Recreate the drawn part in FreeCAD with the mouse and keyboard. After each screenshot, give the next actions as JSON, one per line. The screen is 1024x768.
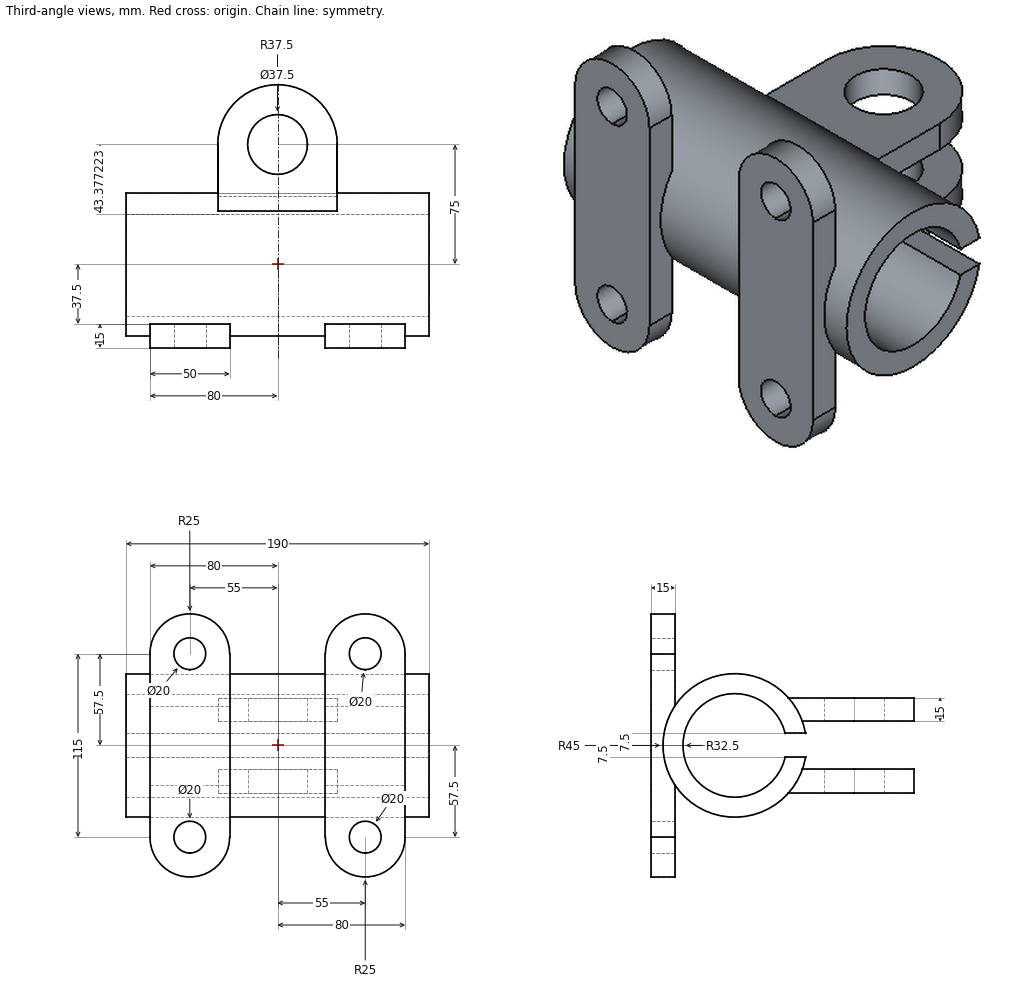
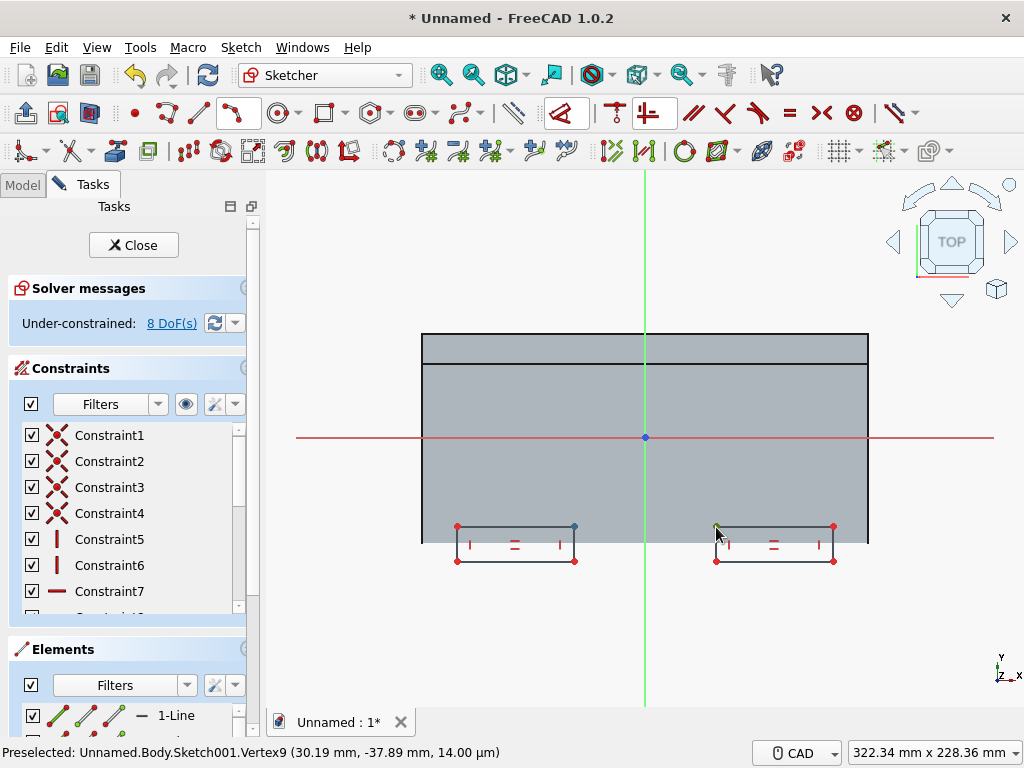
{"action": "left_click", "coordinate": [645, 645]}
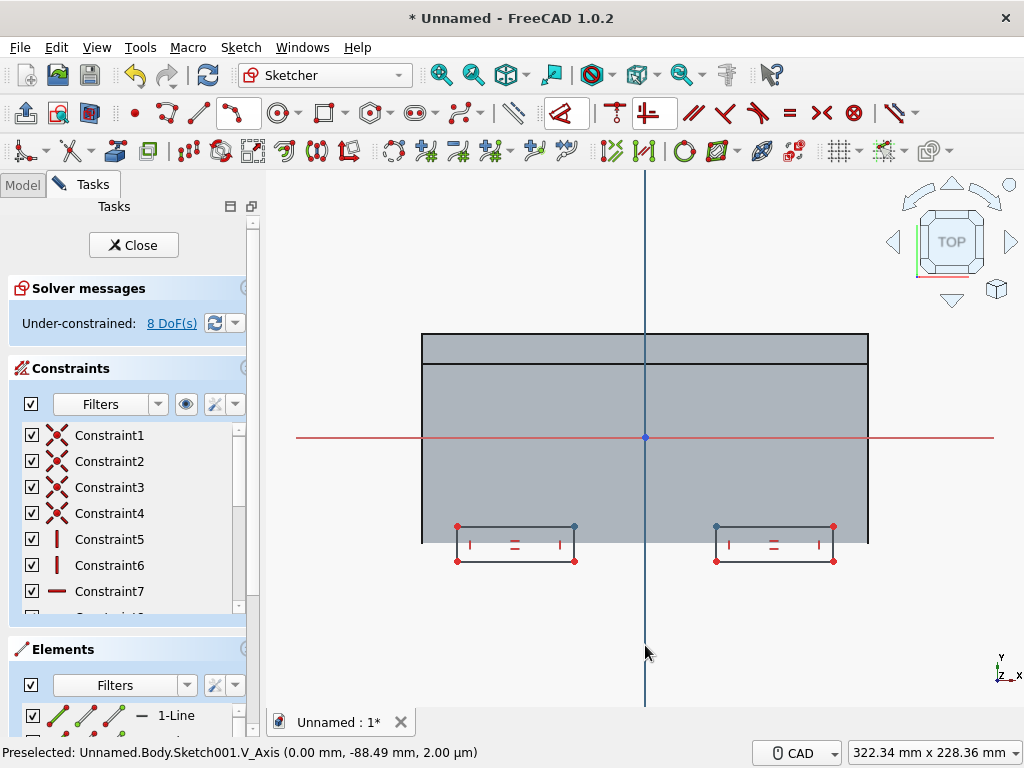
{"action": "left_click", "coordinate": [822, 114]}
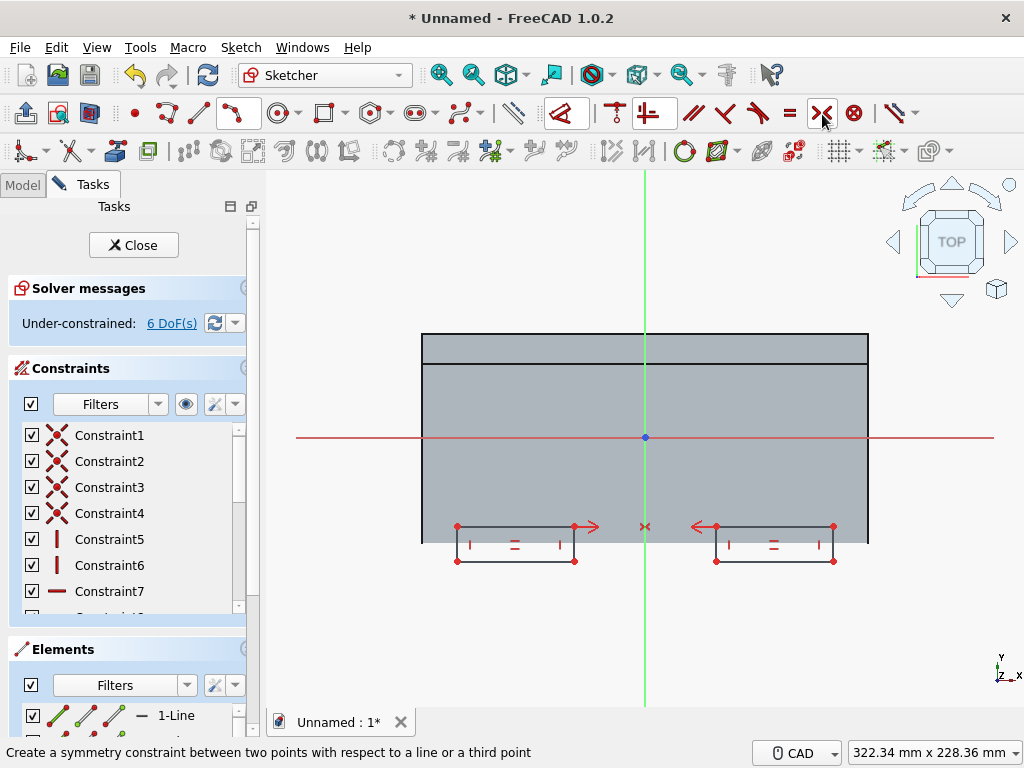
{"action": "left_click", "coordinate": [457, 562]}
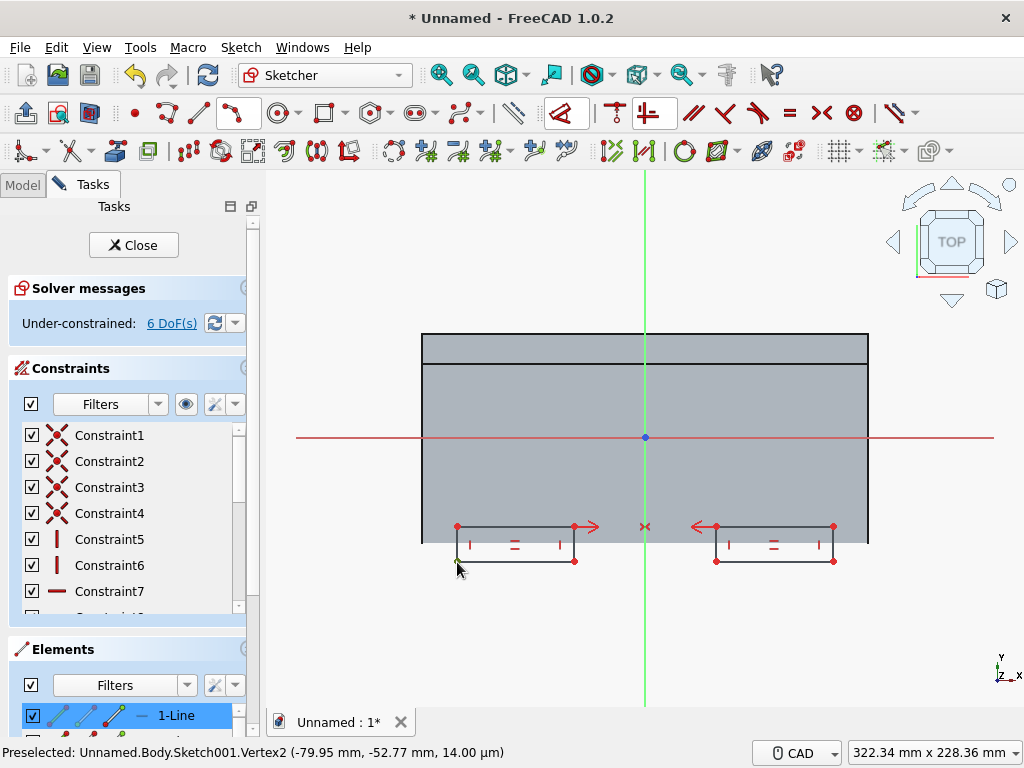
{"action": "left_click", "coordinate": [833, 562]}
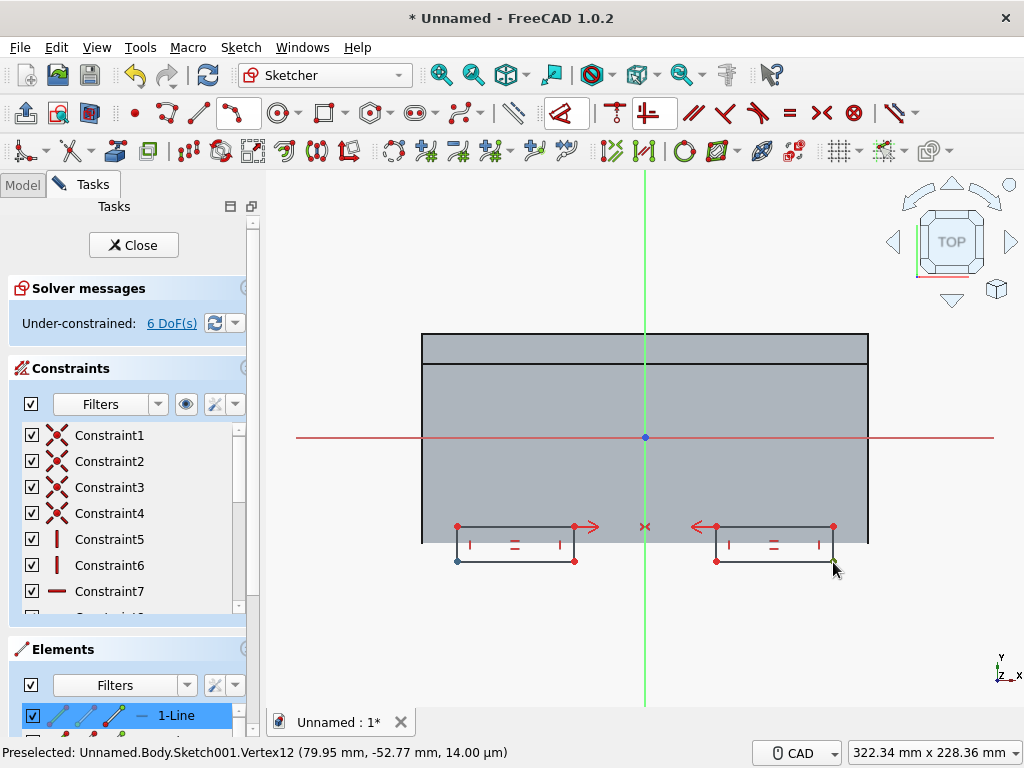
{"action": "left_click", "coordinate": [645, 645]}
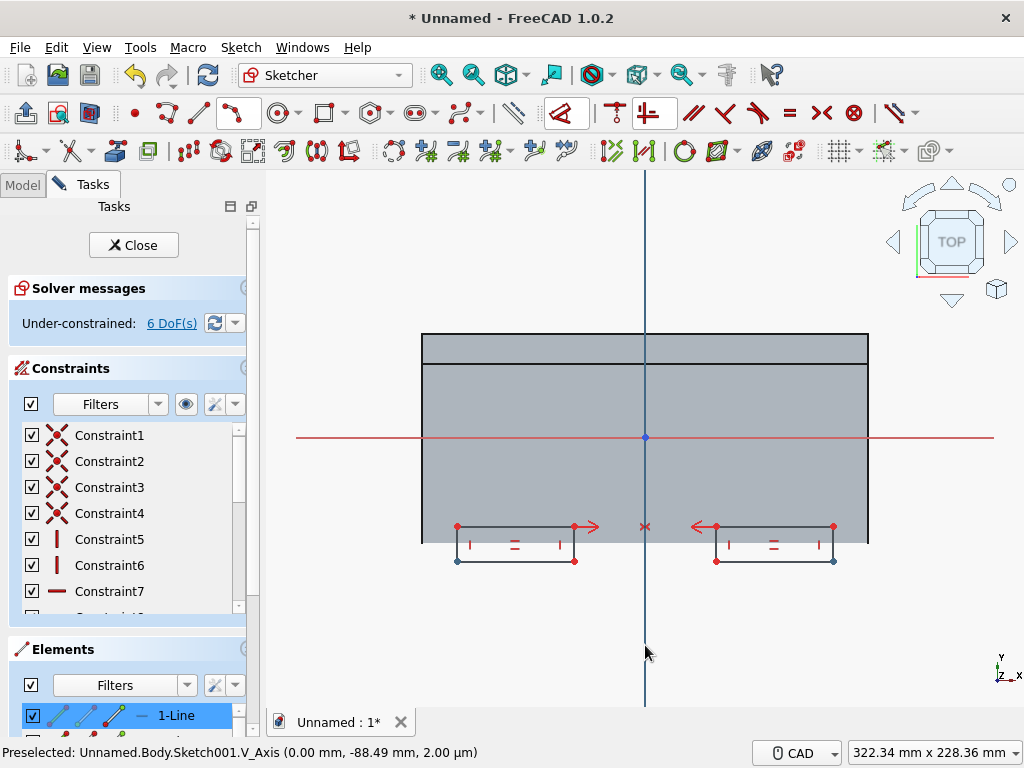
{"action": "left_click", "coordinate": [822, 114]}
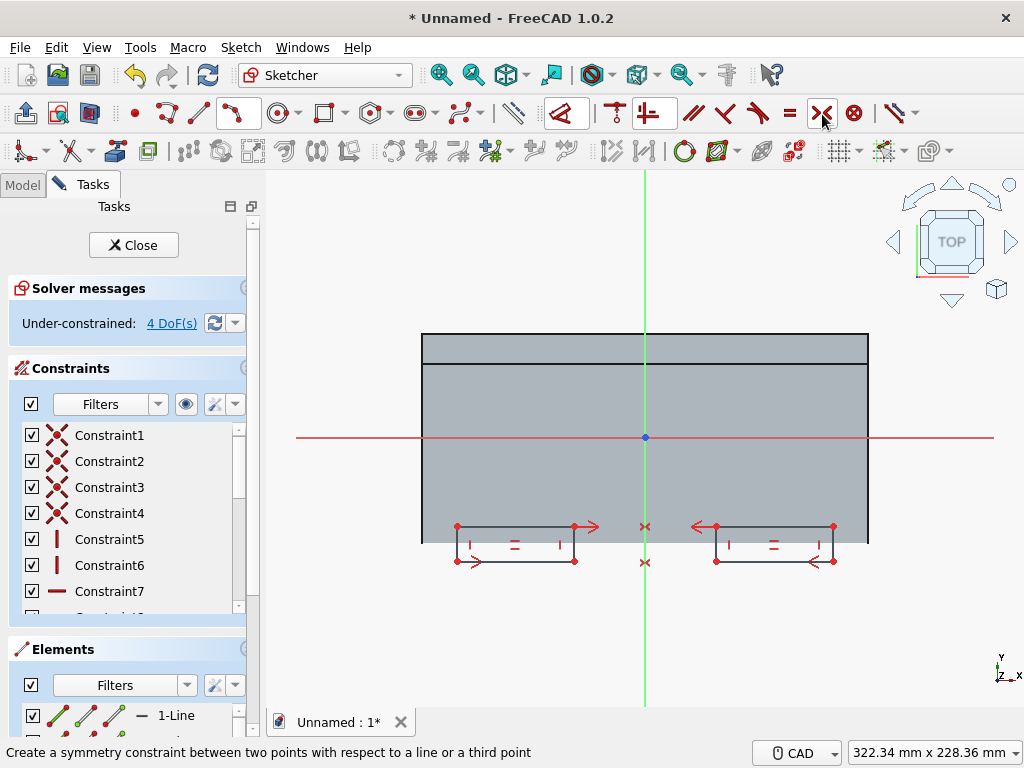
{"action": "scroll", "coordinate": [457, 537], "scroll_direction": "up", "scroll_amount": 2}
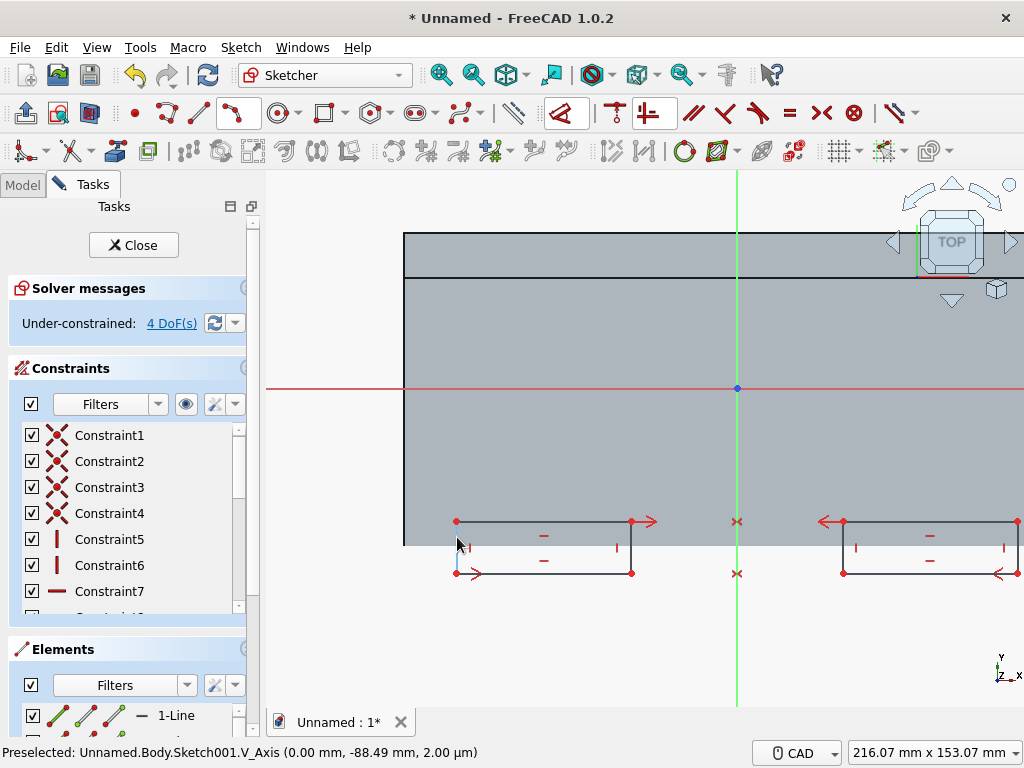
{"action": "left_click", "coordinate": [457, 537]}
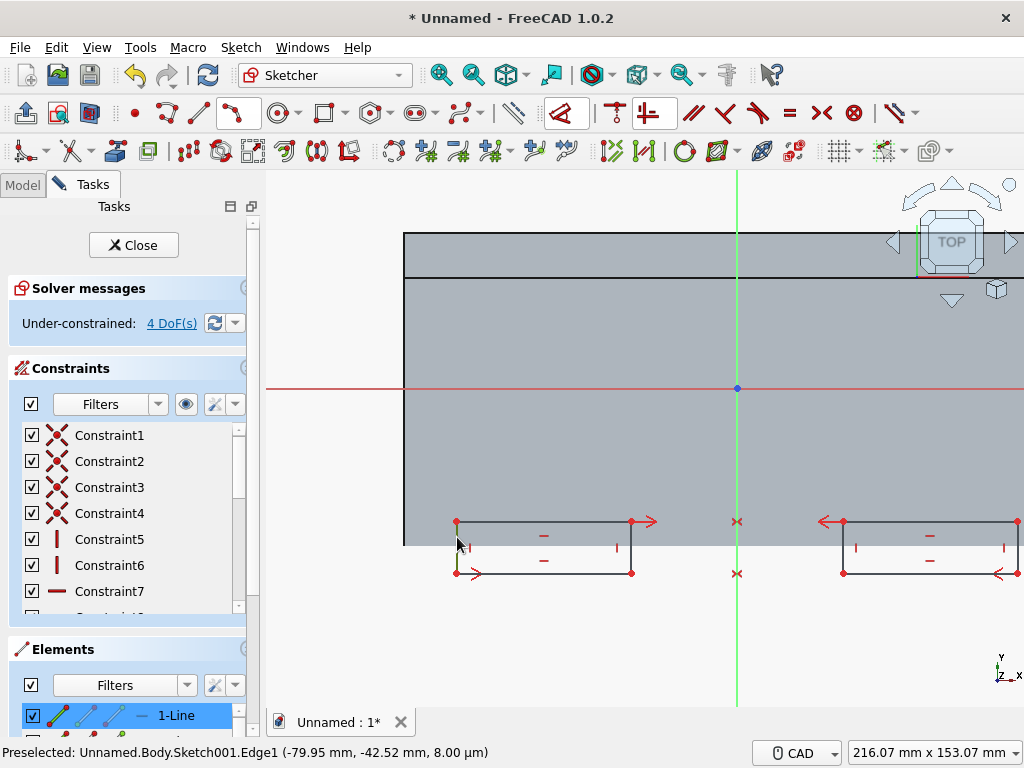
{"action": "left_click", "coordinate": [584, 114]}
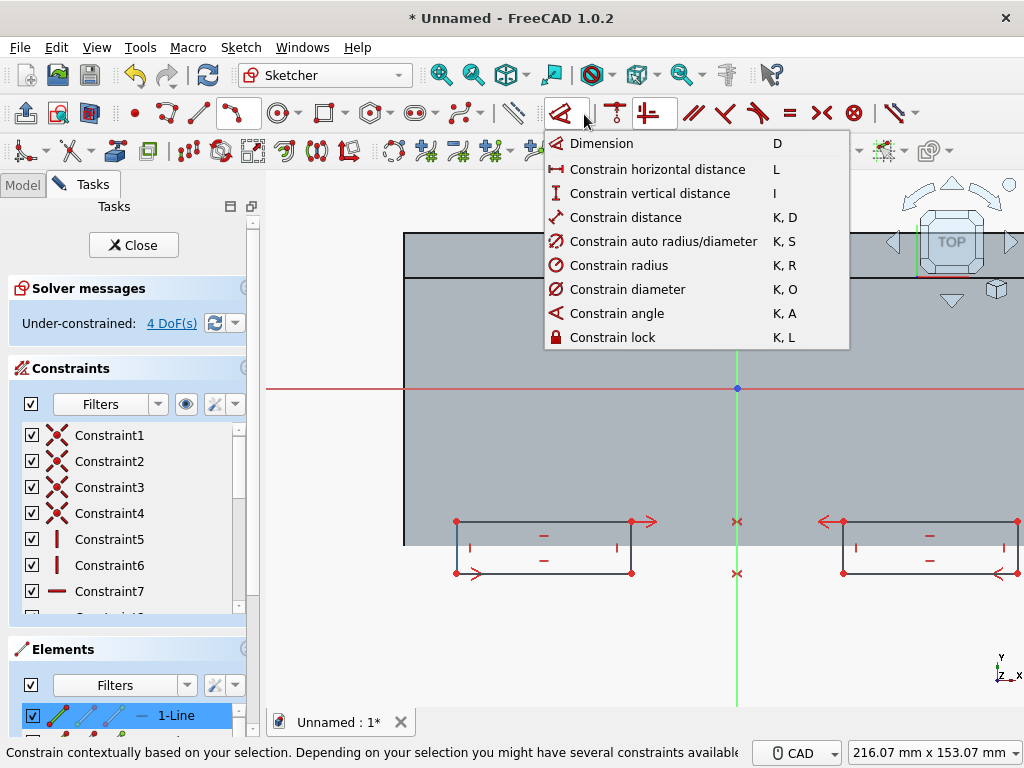
{"action": "left_click", "coordinate": [697, 193]}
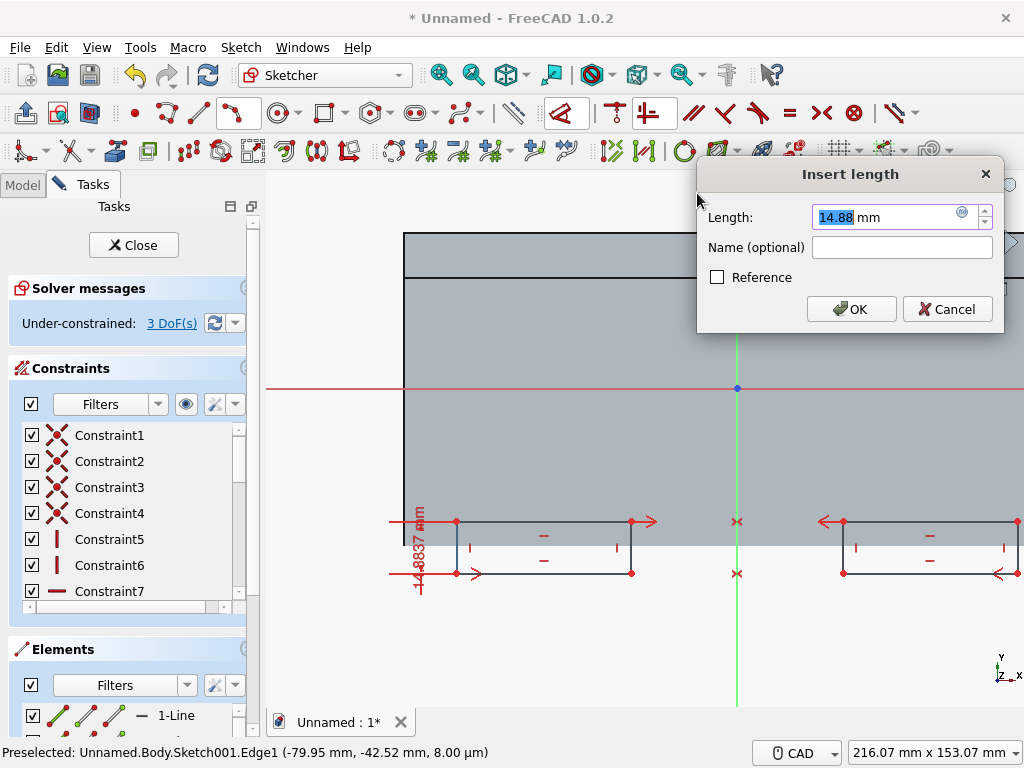
{"action": "type", "text": "15"}
{"action": "key", "text": "Return"}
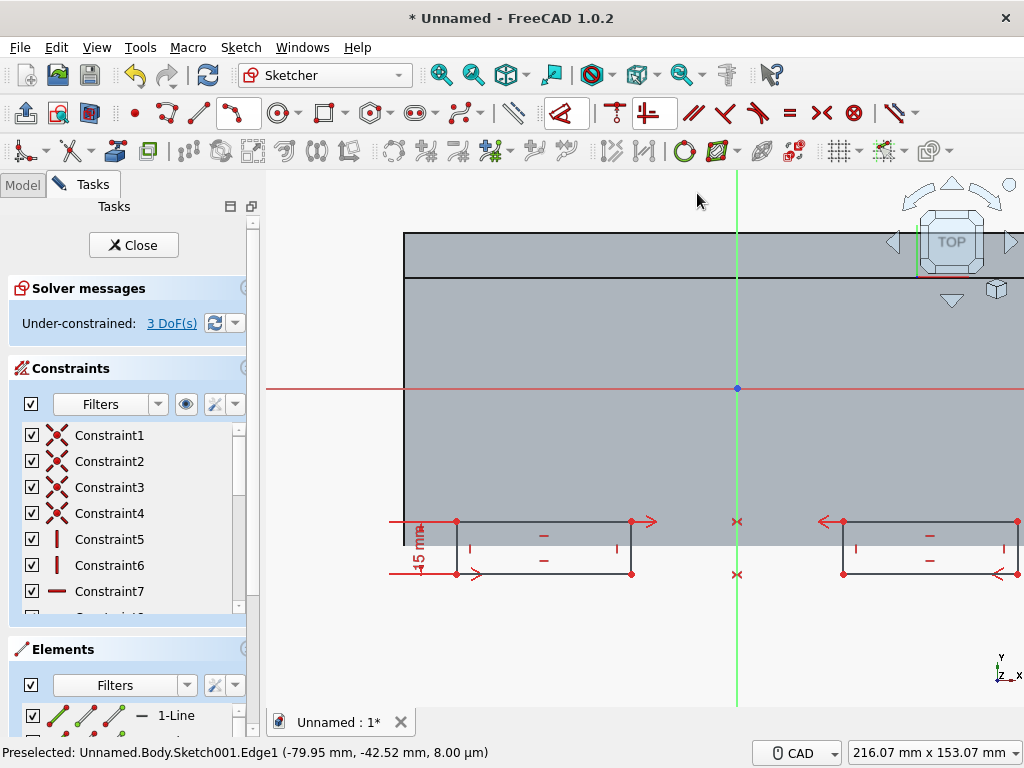
{"action": "left_click", "coordinate": [509, 574]}